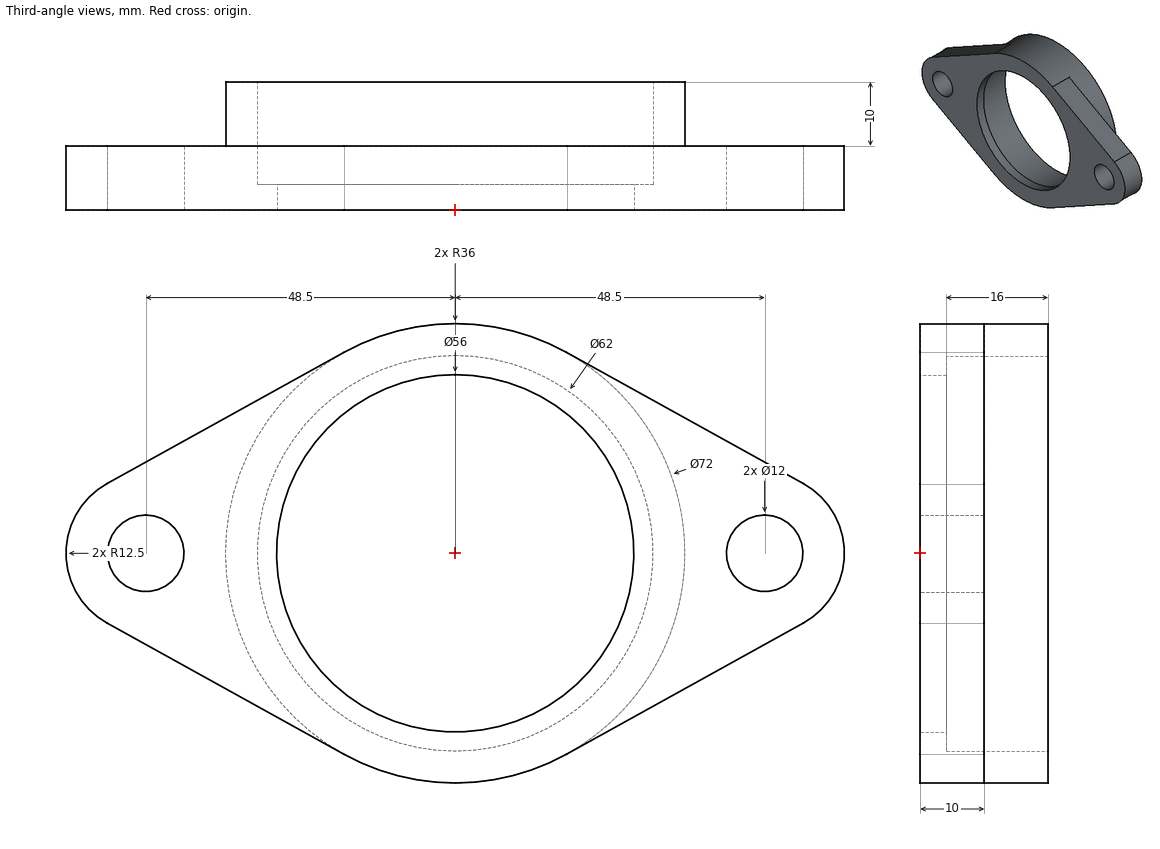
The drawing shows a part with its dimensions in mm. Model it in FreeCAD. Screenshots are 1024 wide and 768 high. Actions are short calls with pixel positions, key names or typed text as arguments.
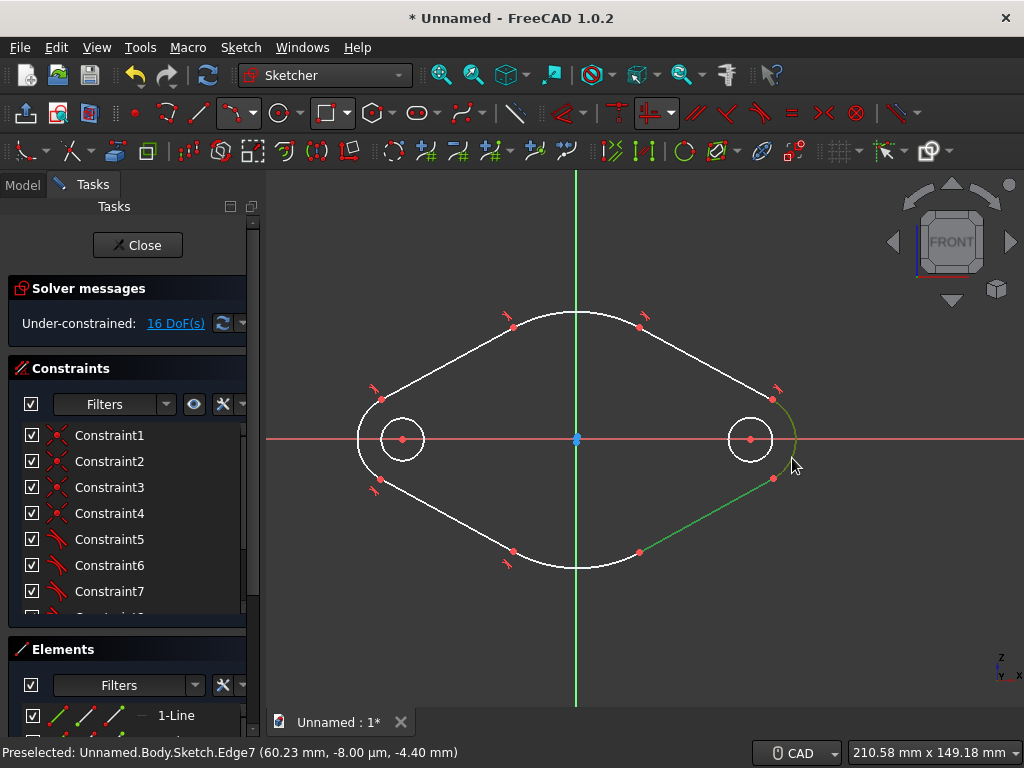
click(760, 114)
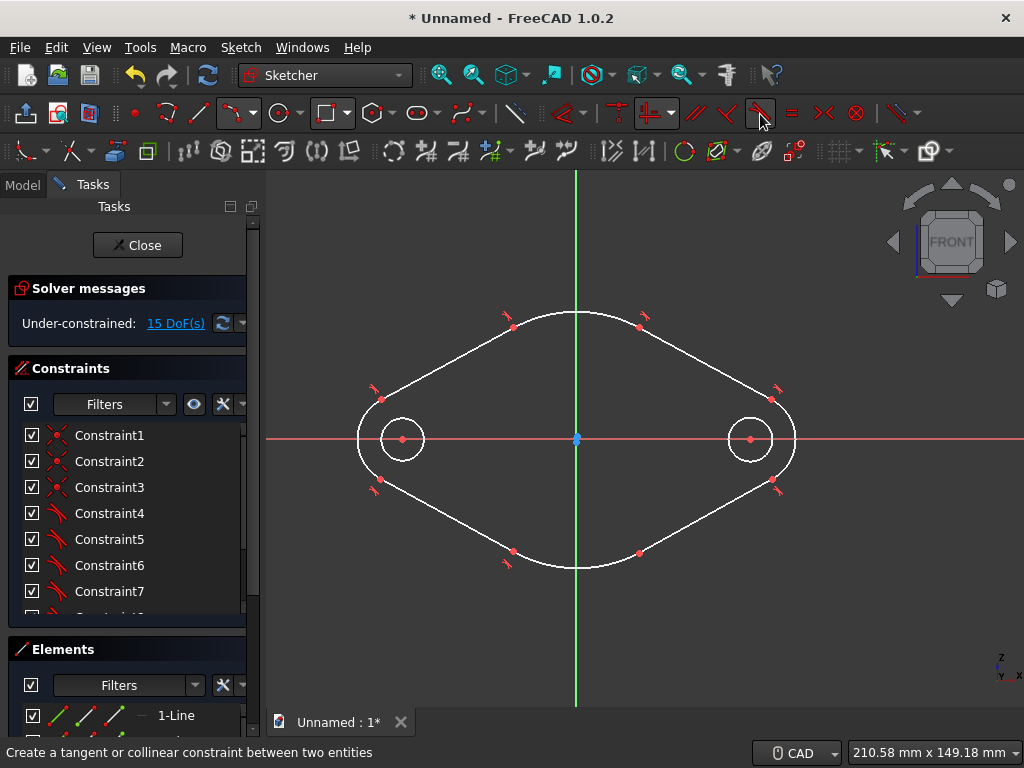
click(732, 501)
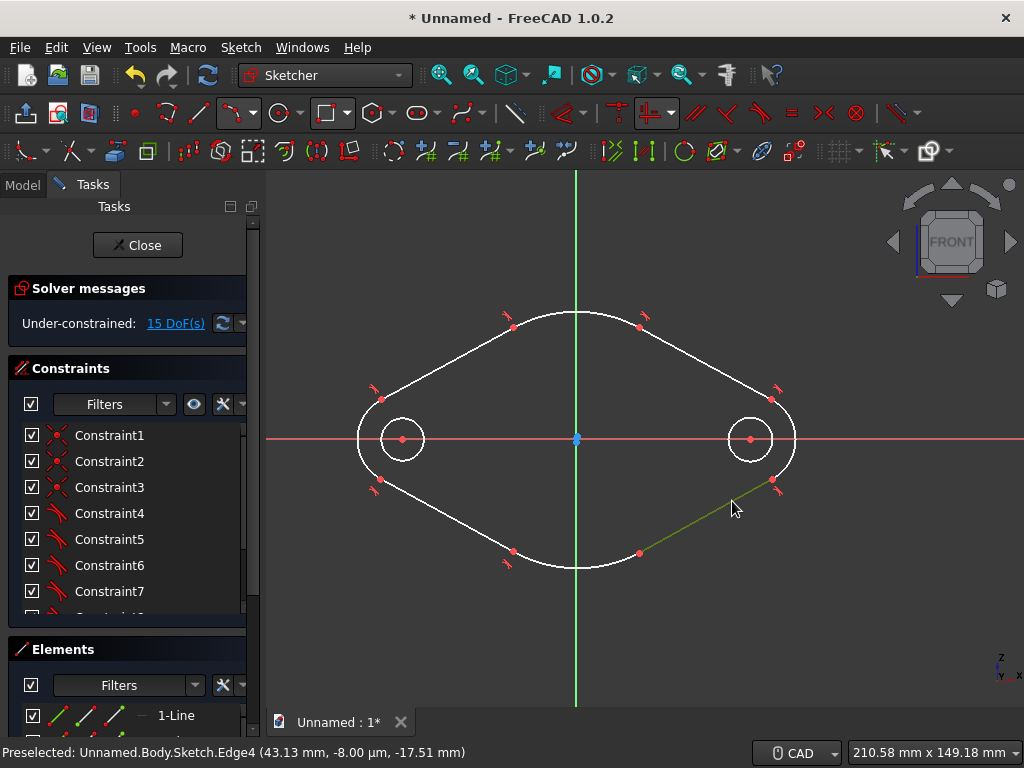
click(551, 565)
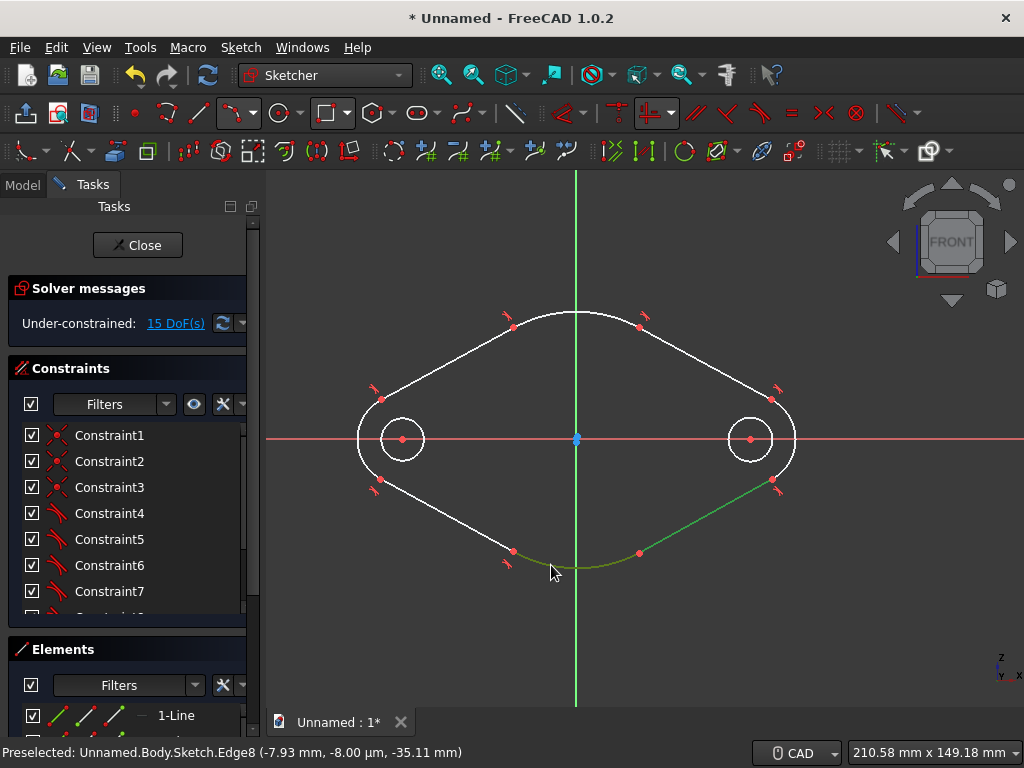
click(760, 114)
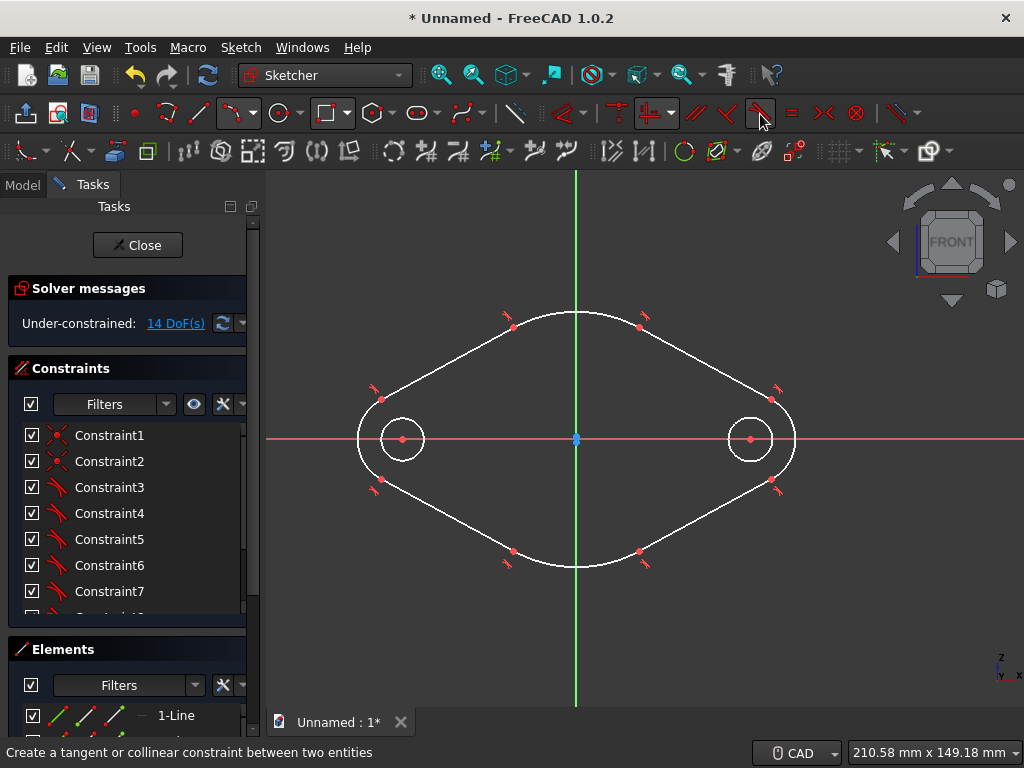
click(602, 314)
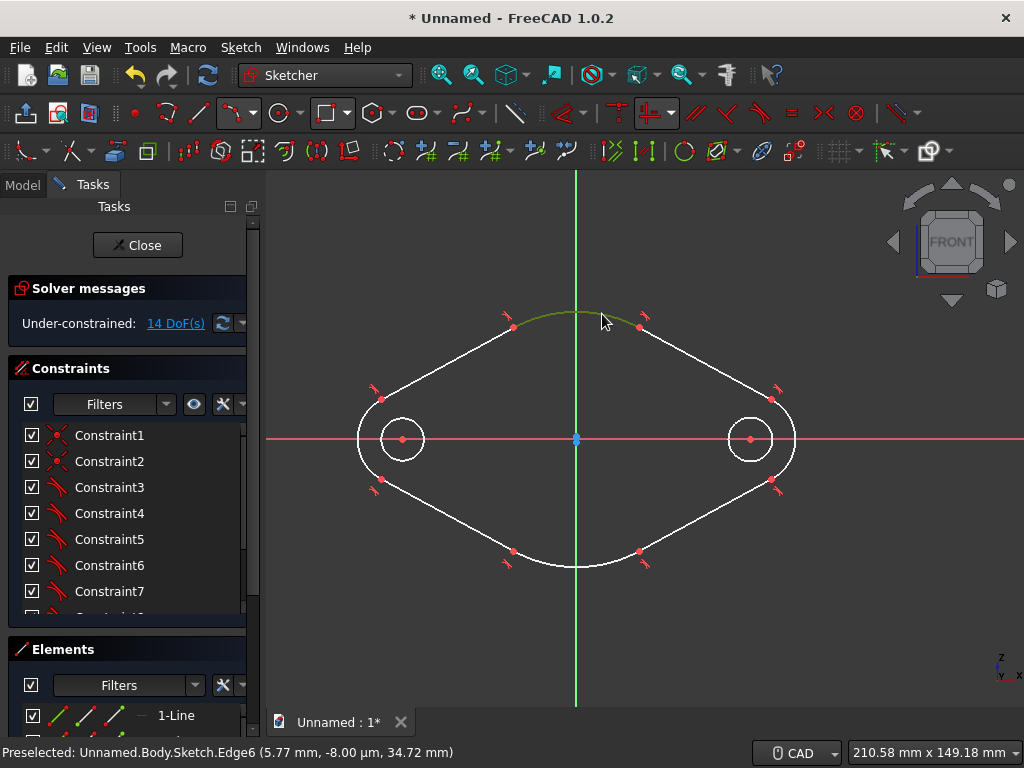
click(551, 565)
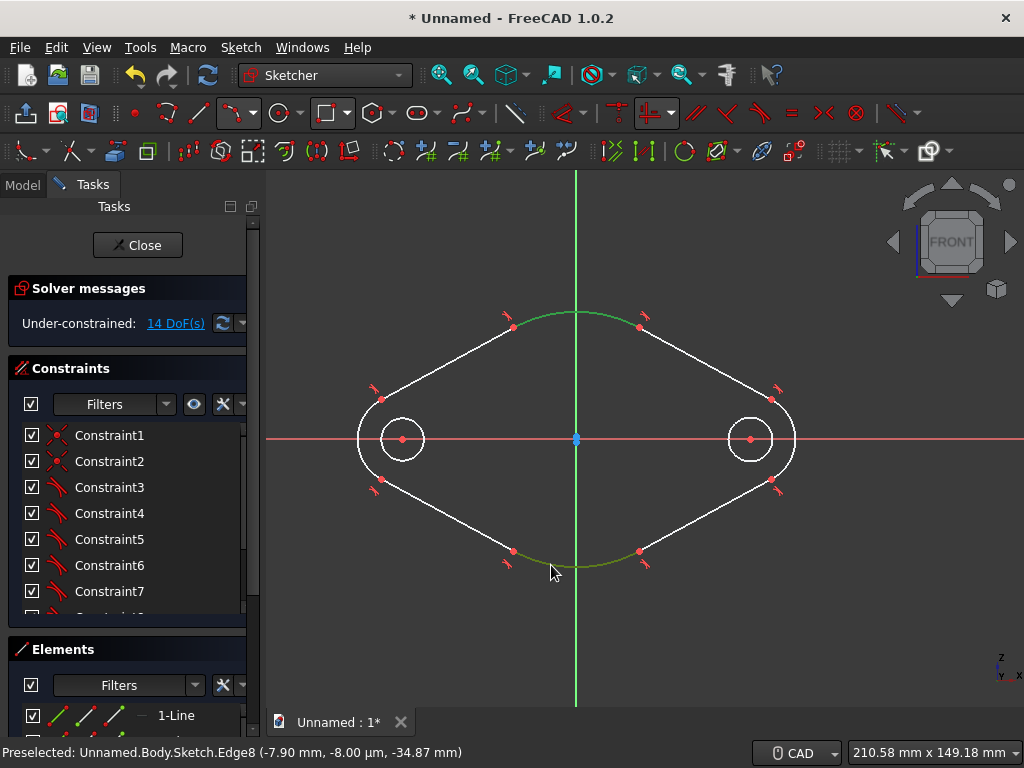
click(618, 114)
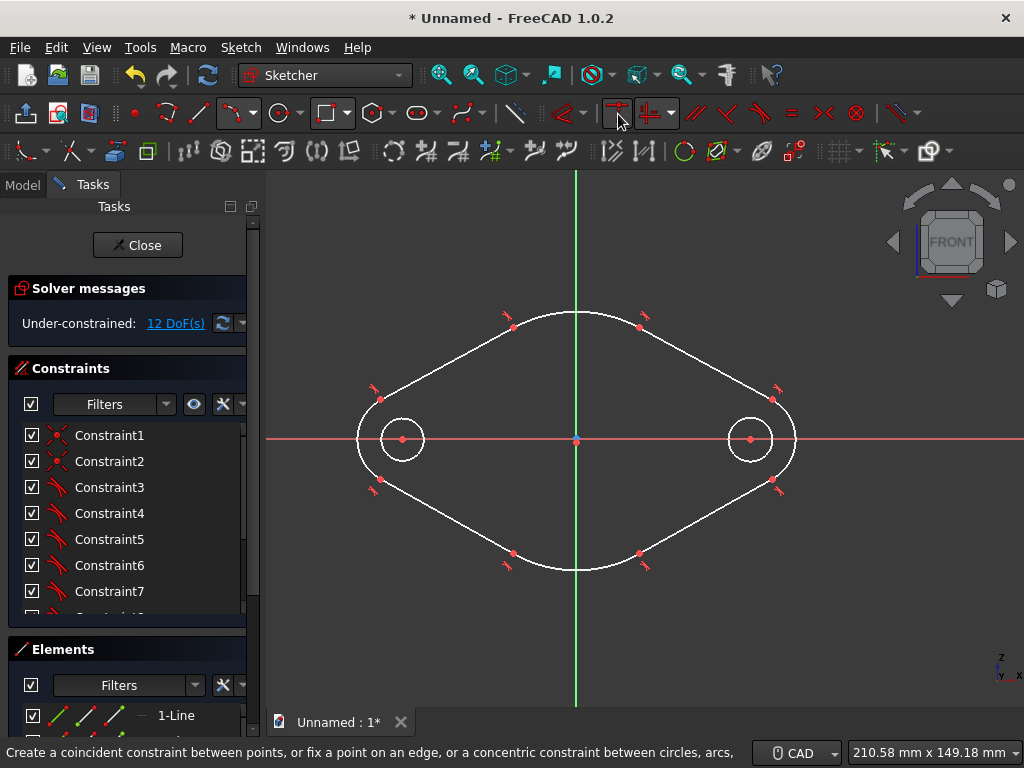
scroll(577, 441, up, 4)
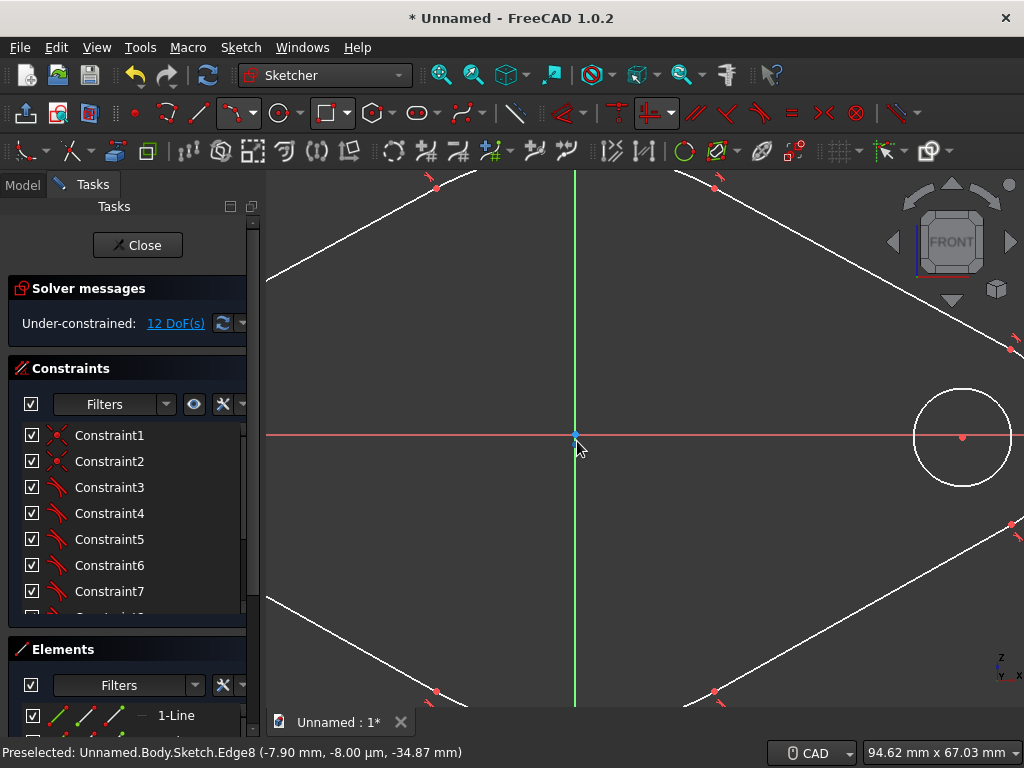
drag(565, 425, 585, 454)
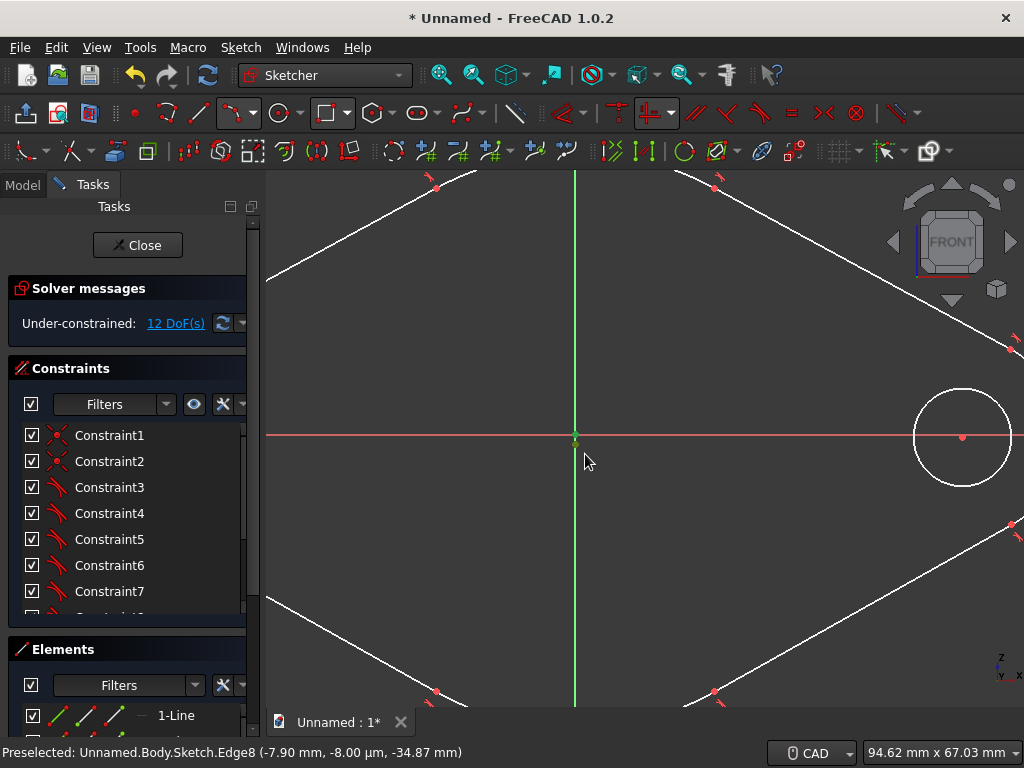
click(618, 114)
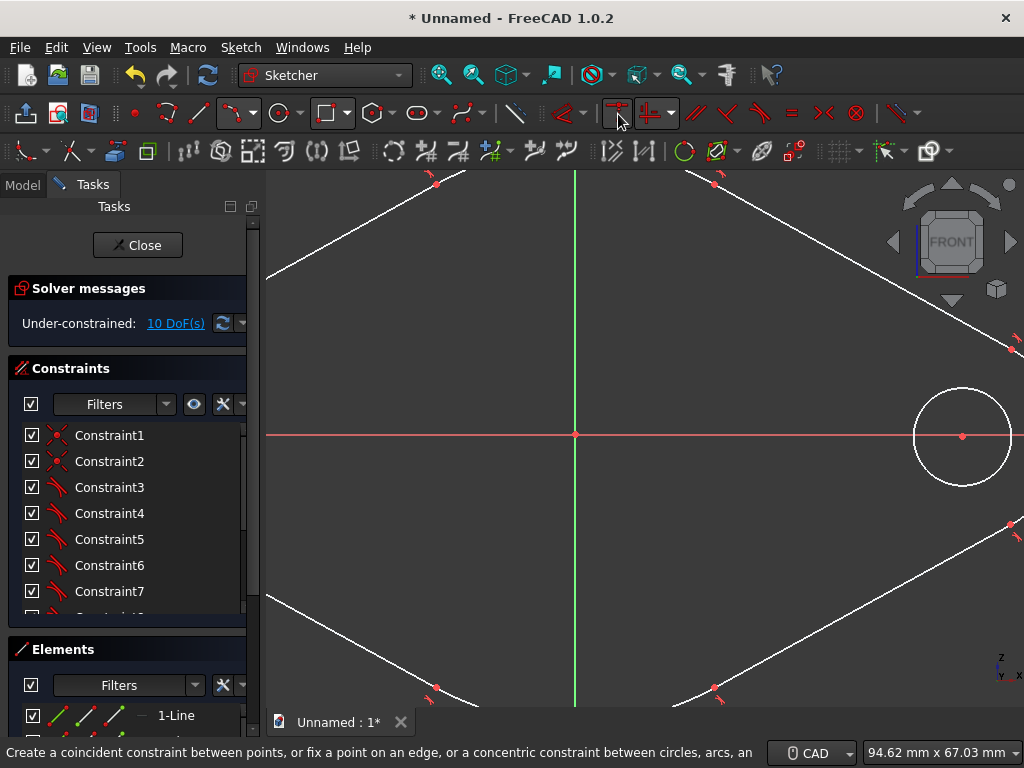
scroll(577, 442, down, 4)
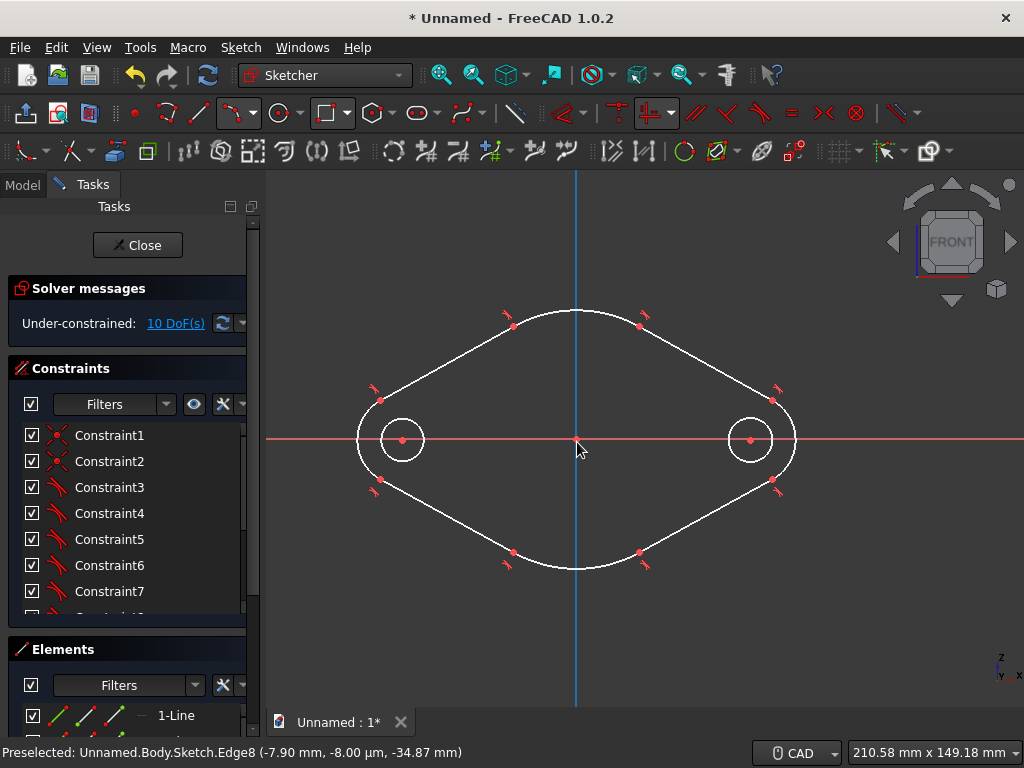
click(361, 421)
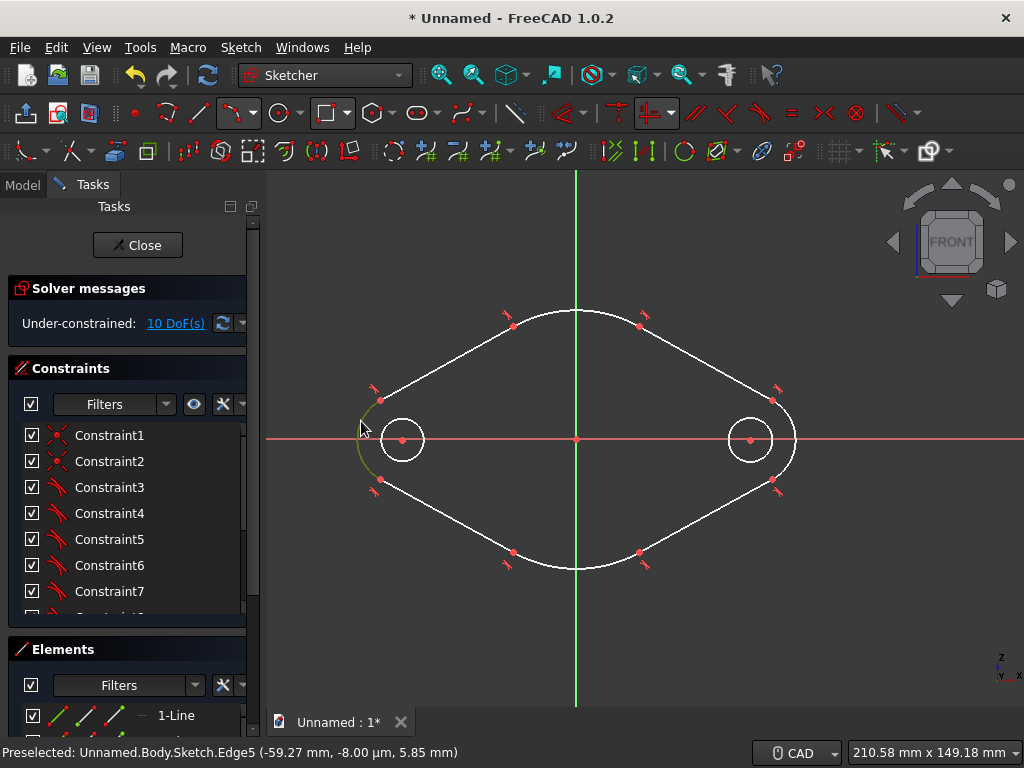
click(791, 459)